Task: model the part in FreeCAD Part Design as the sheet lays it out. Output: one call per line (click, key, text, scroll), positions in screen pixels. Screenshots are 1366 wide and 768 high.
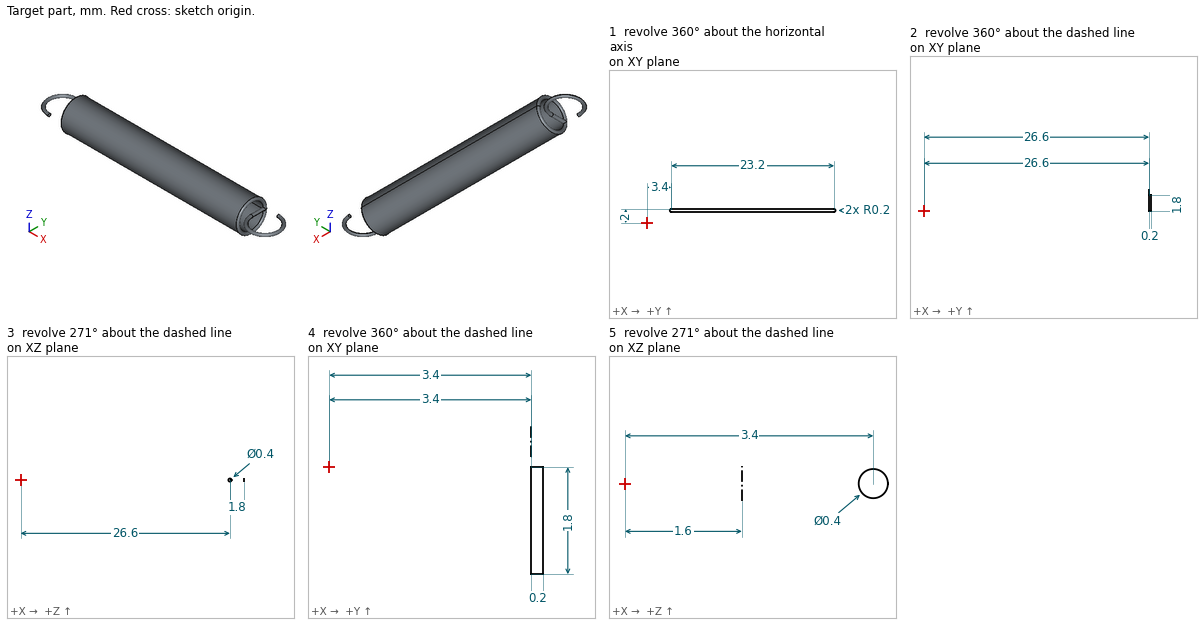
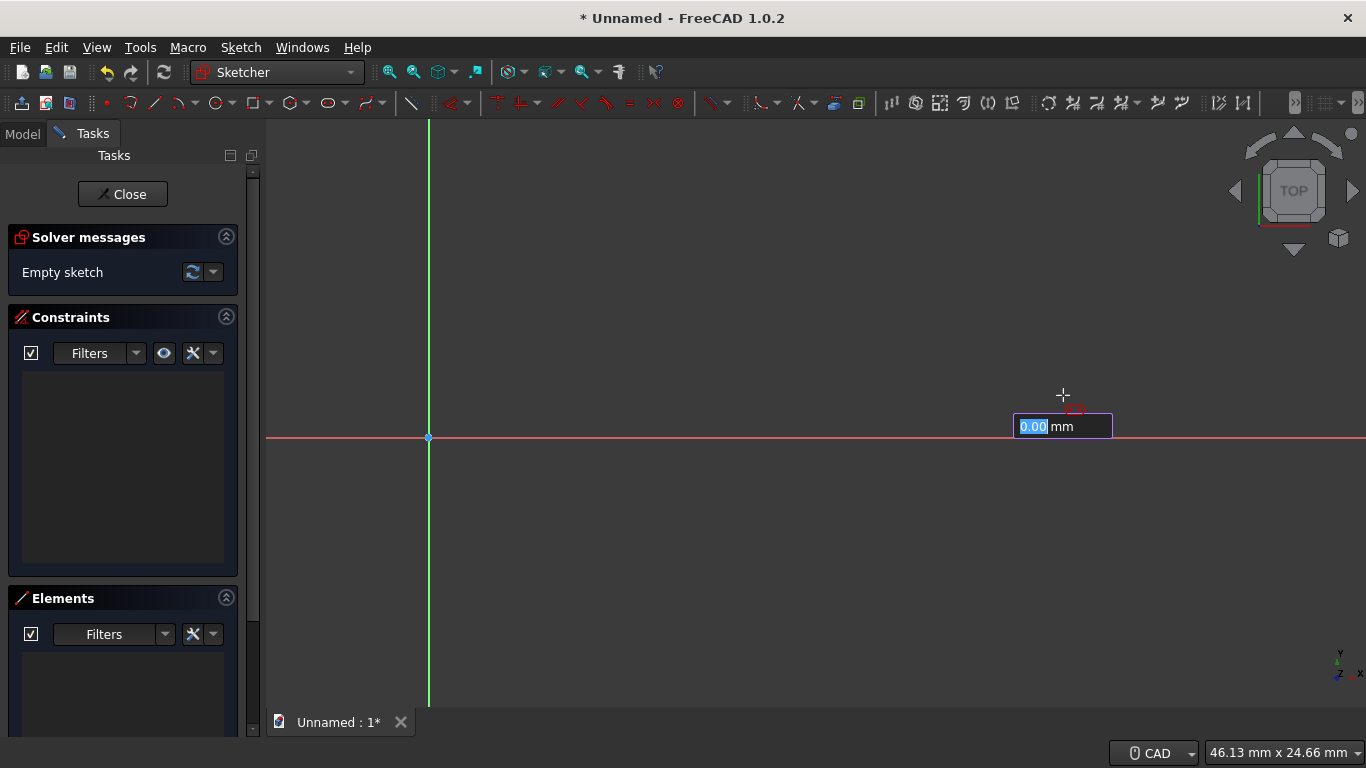
scroll(786, 399, up, 7)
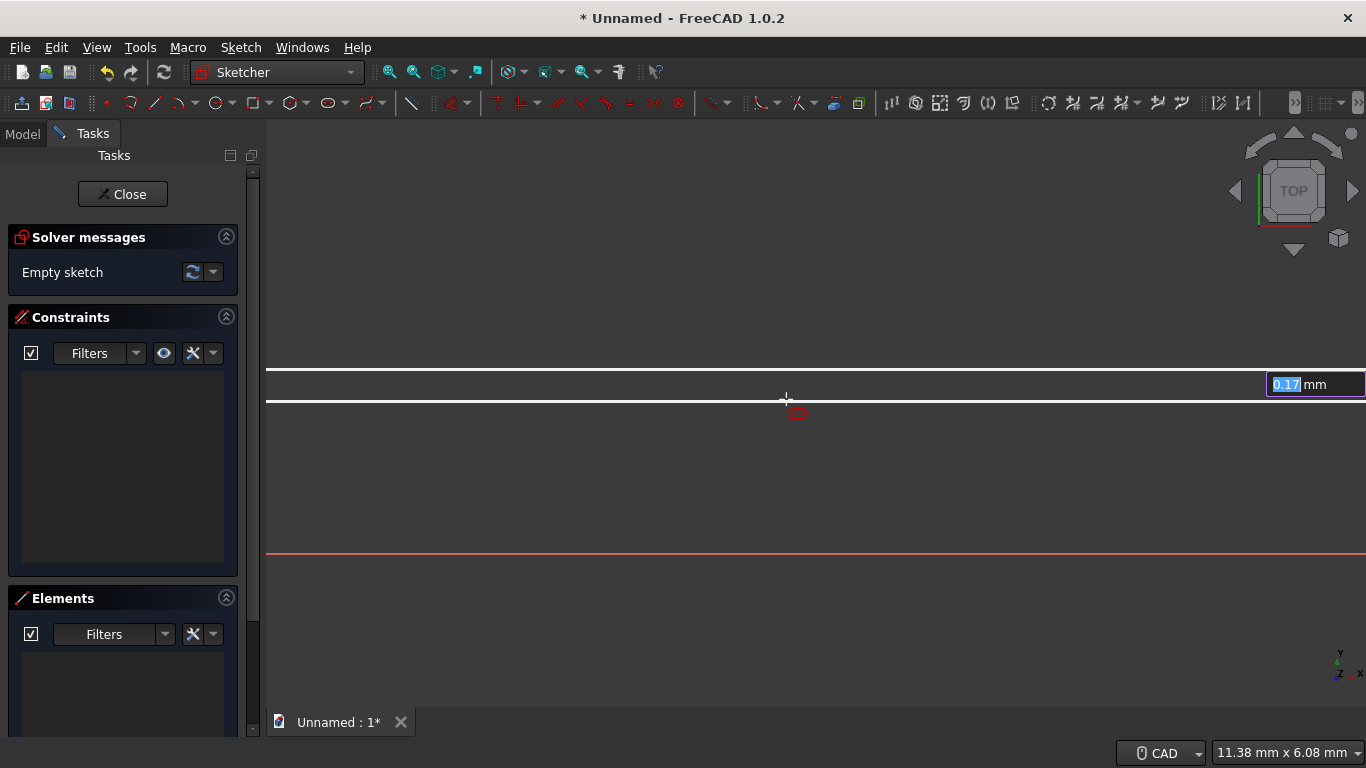
click(785, 399)
key(Escape)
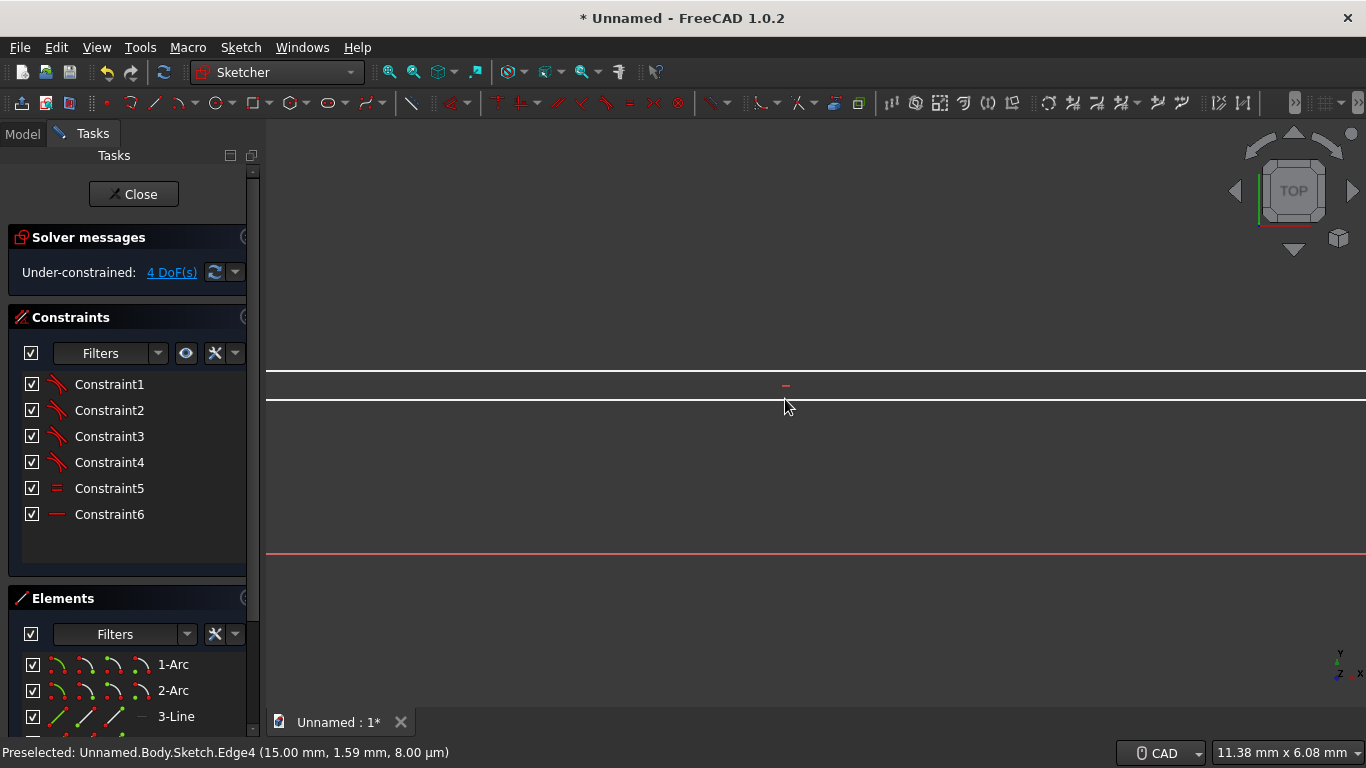
scroll(786, 399, down, 7)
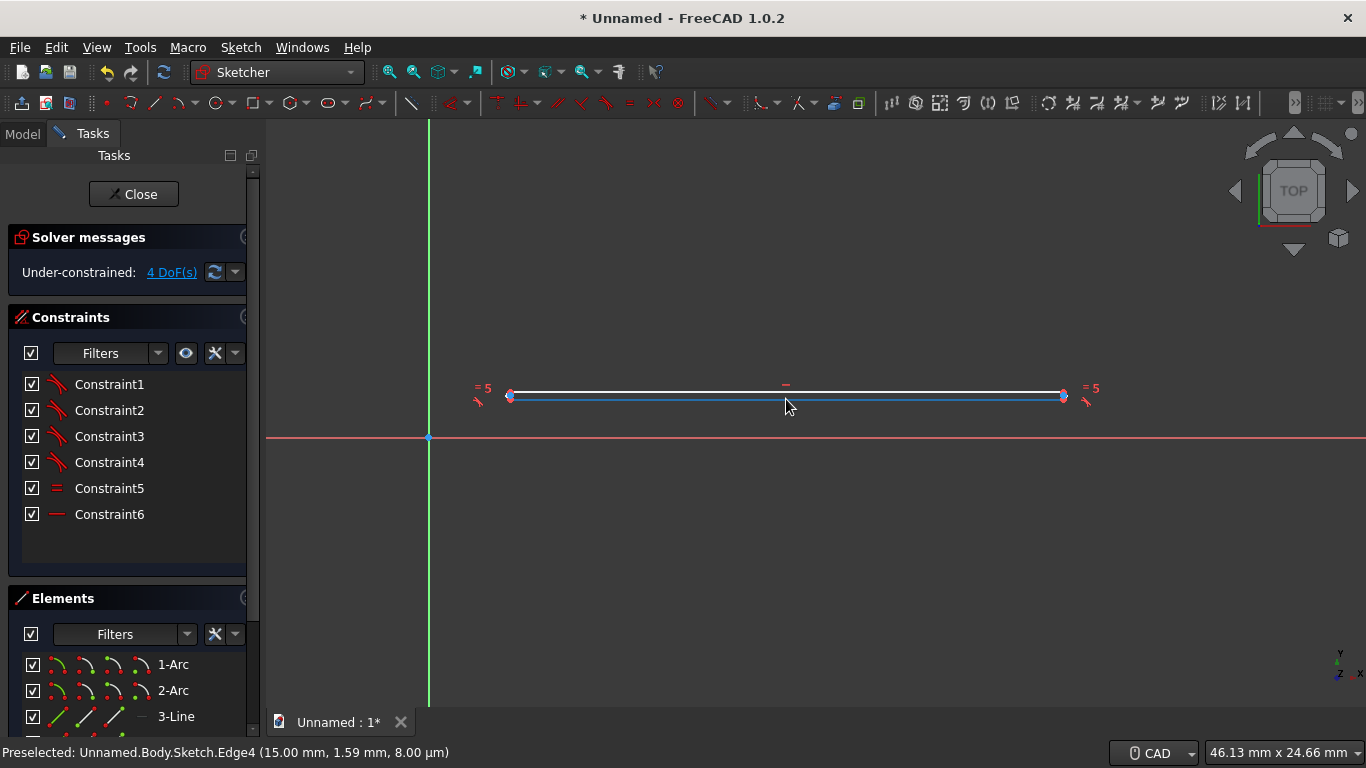
scroll(507, 394, up, 11)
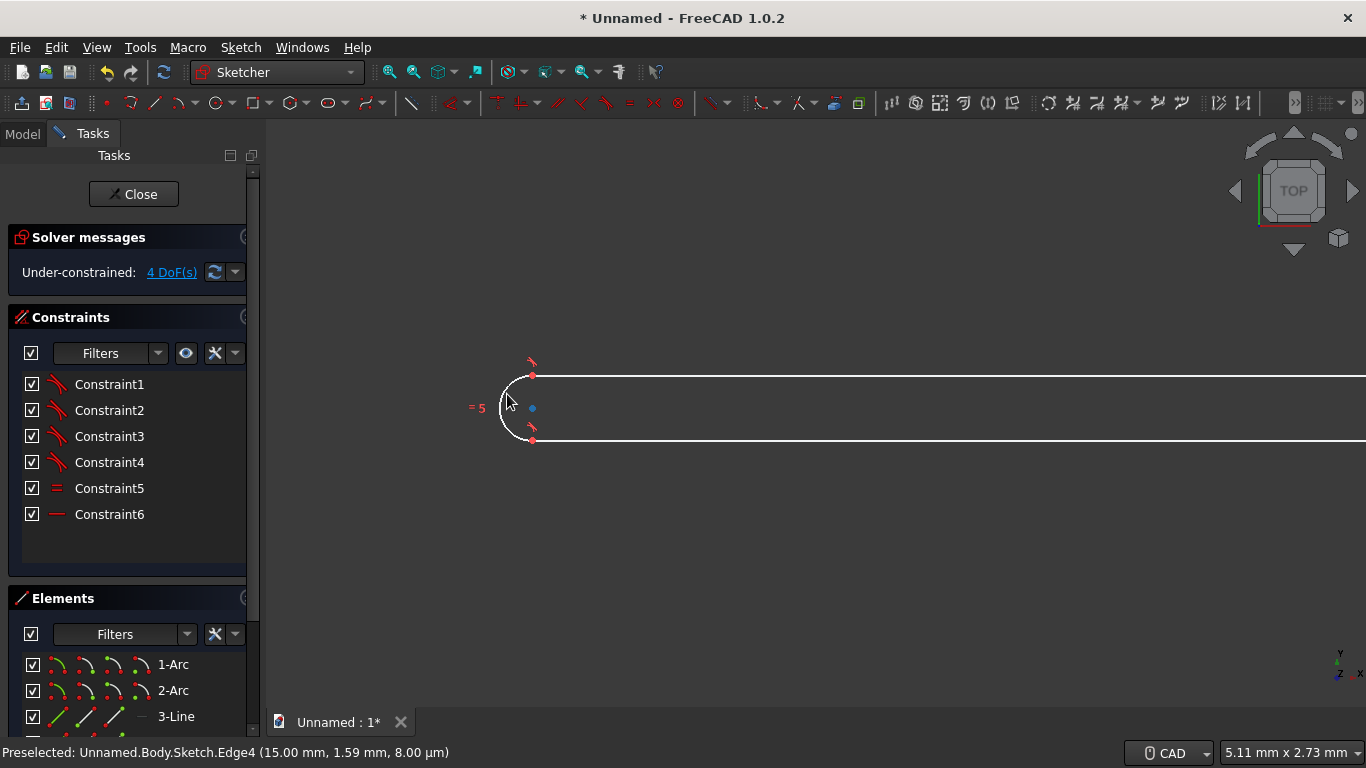
click(506, 389)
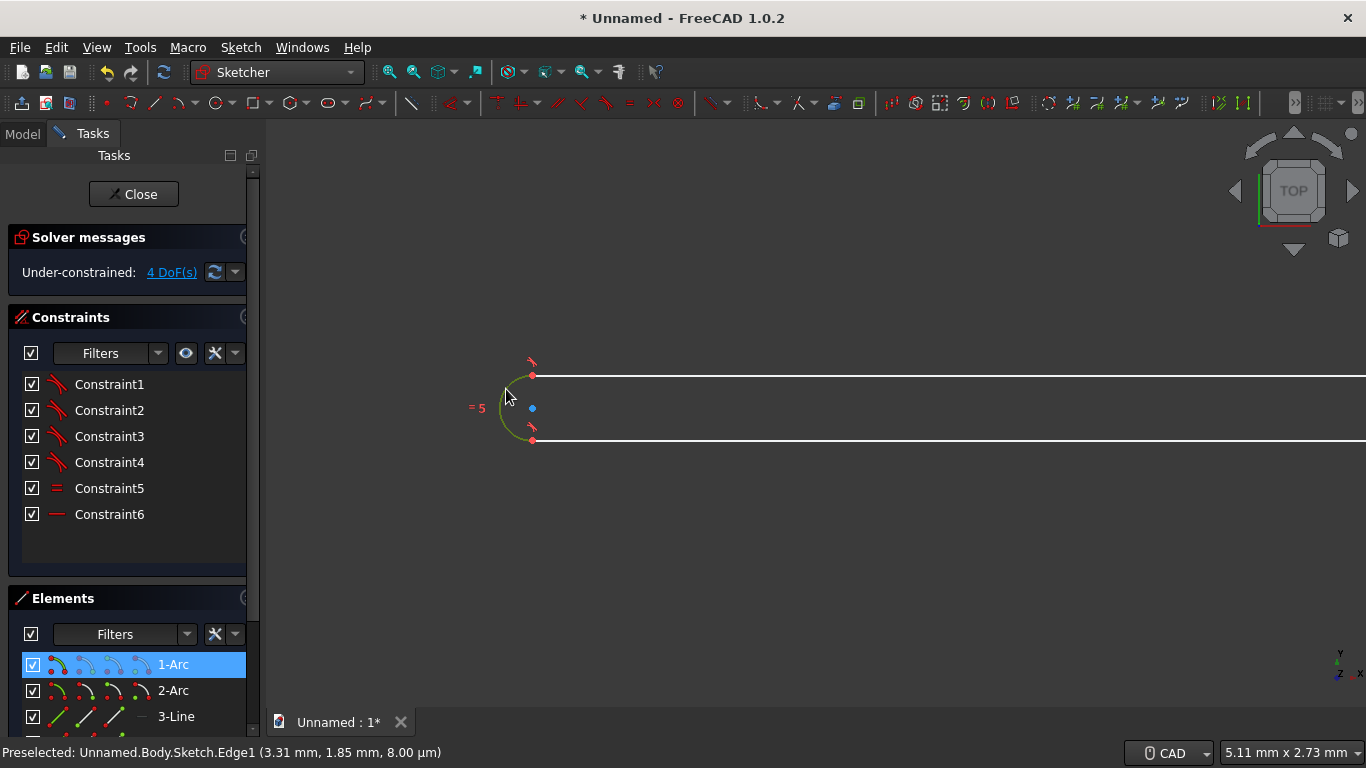
key(k)
key(r)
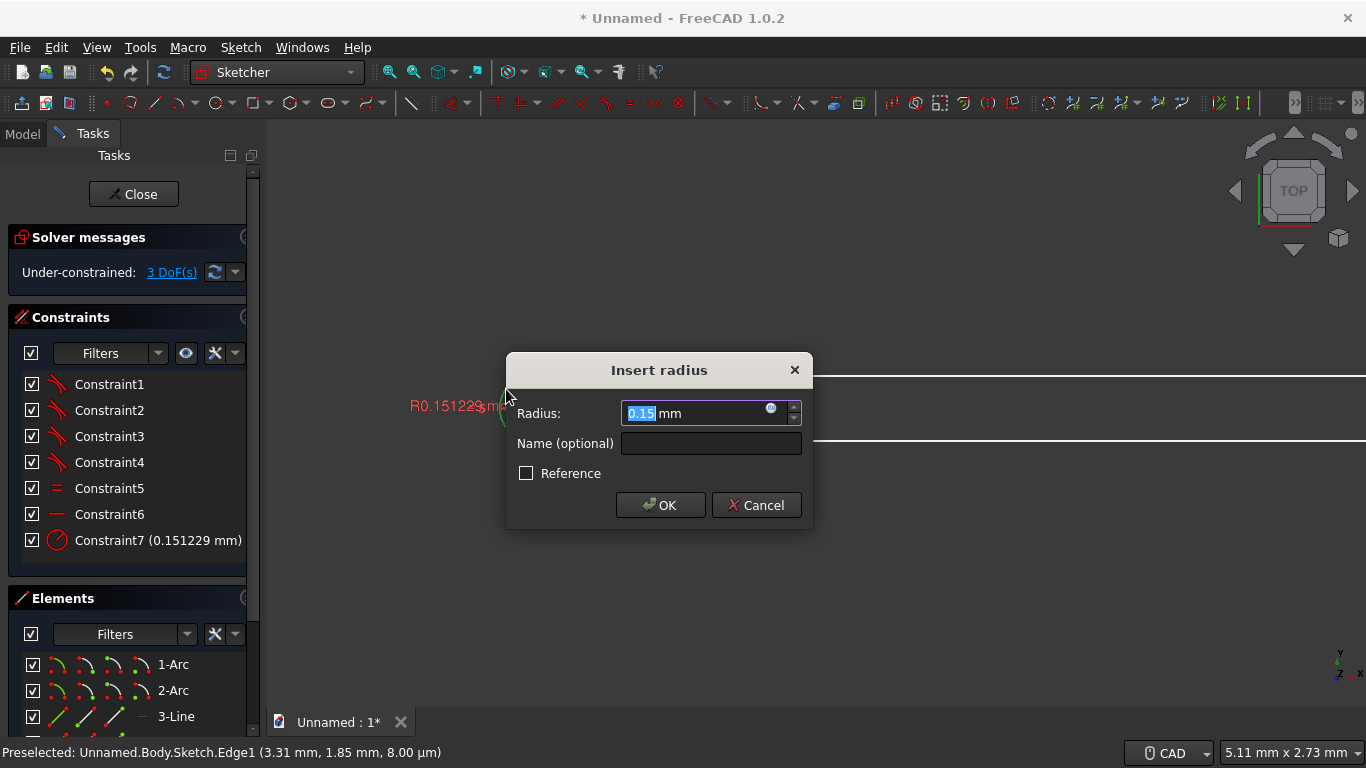
text(0.2)
key(Return)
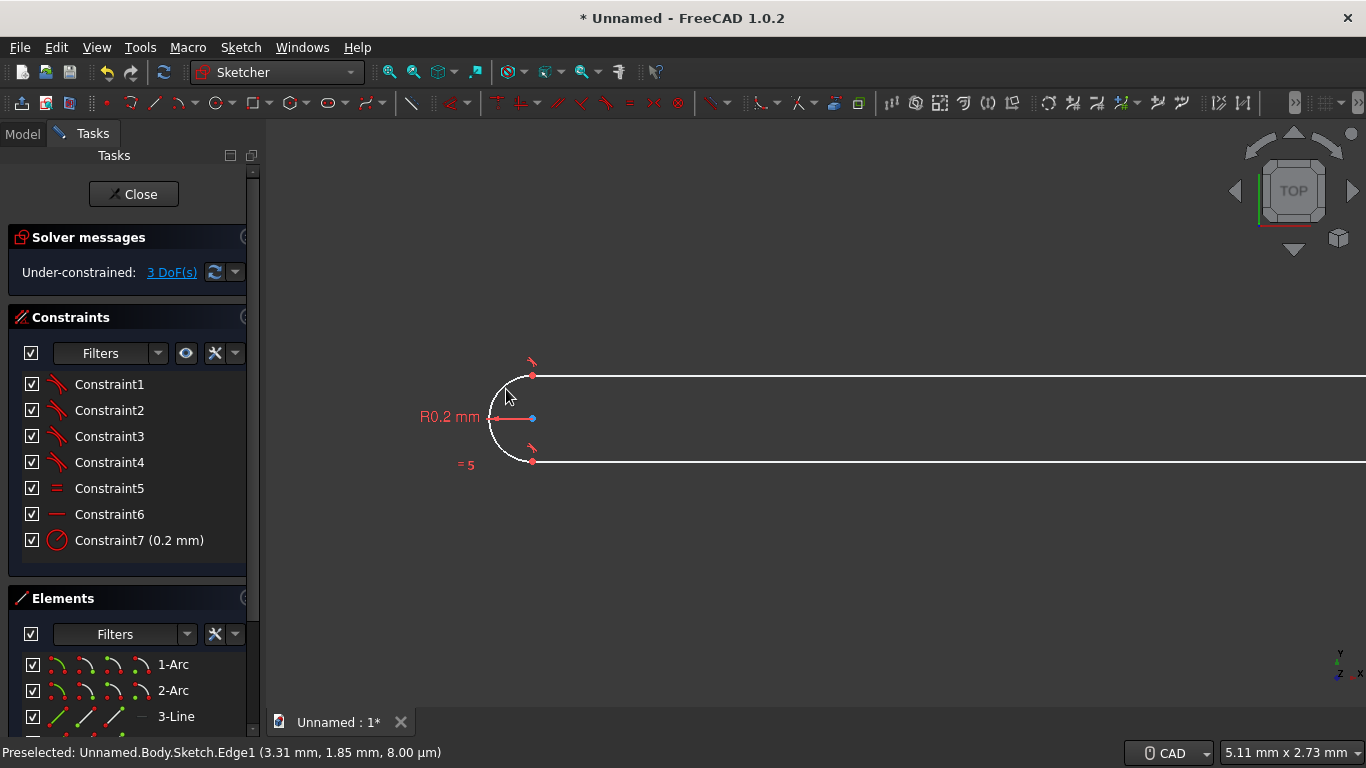
scroll(507, 394, down, 11)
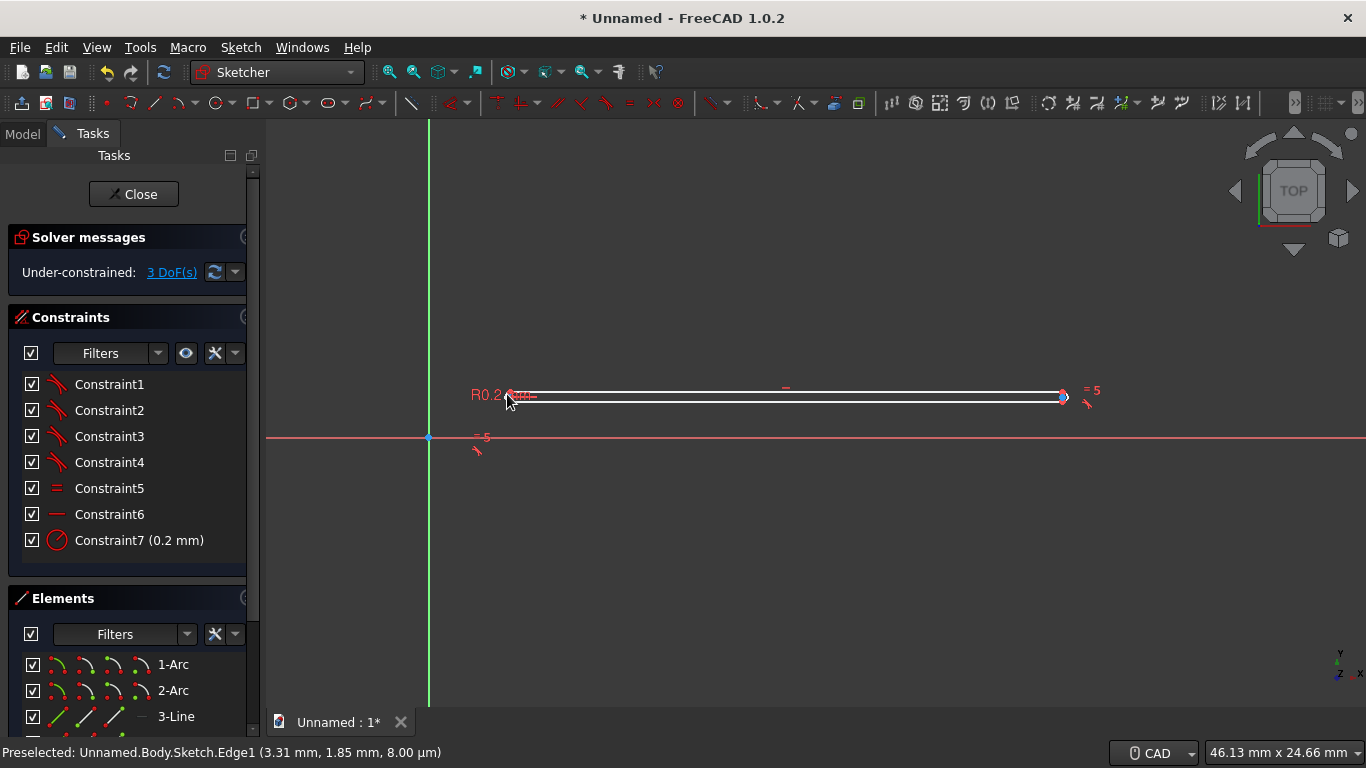
scroll(510, 392, up, 5)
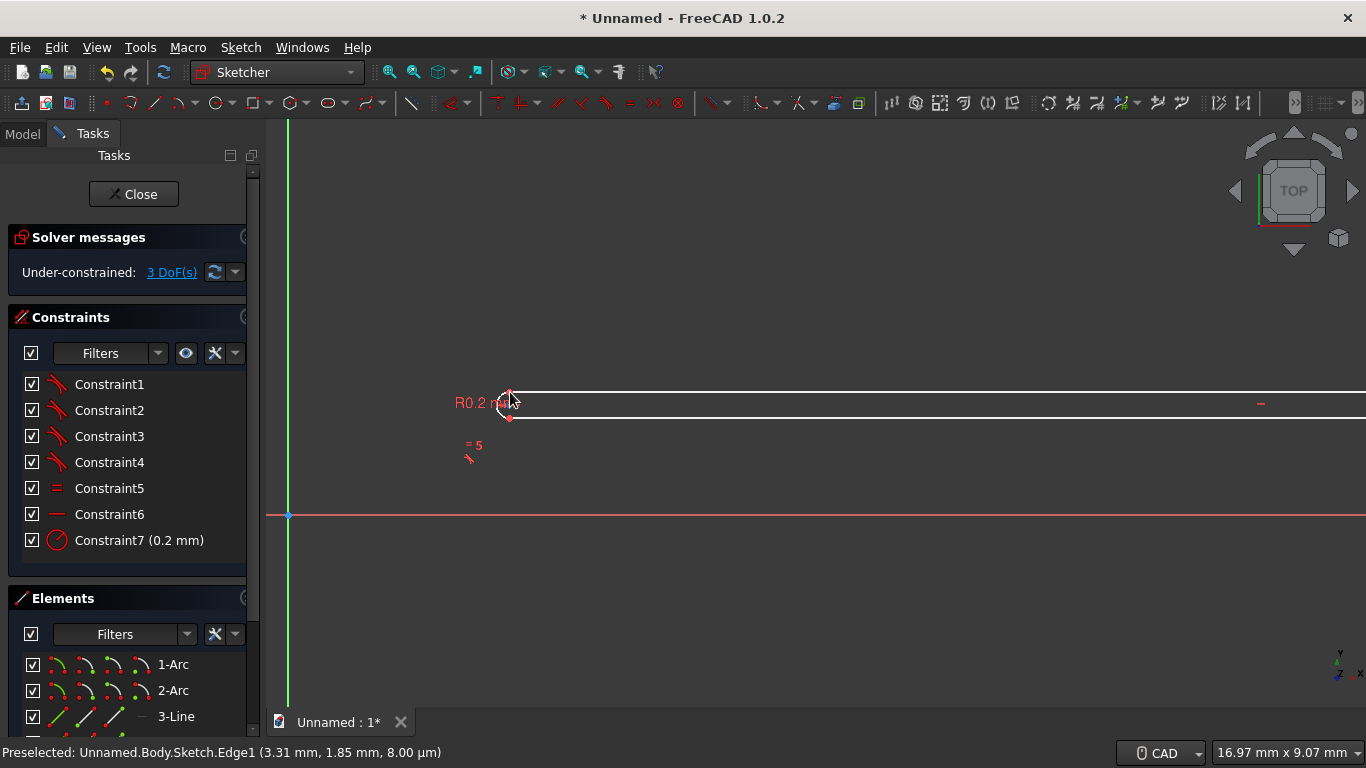
click(510, 392)